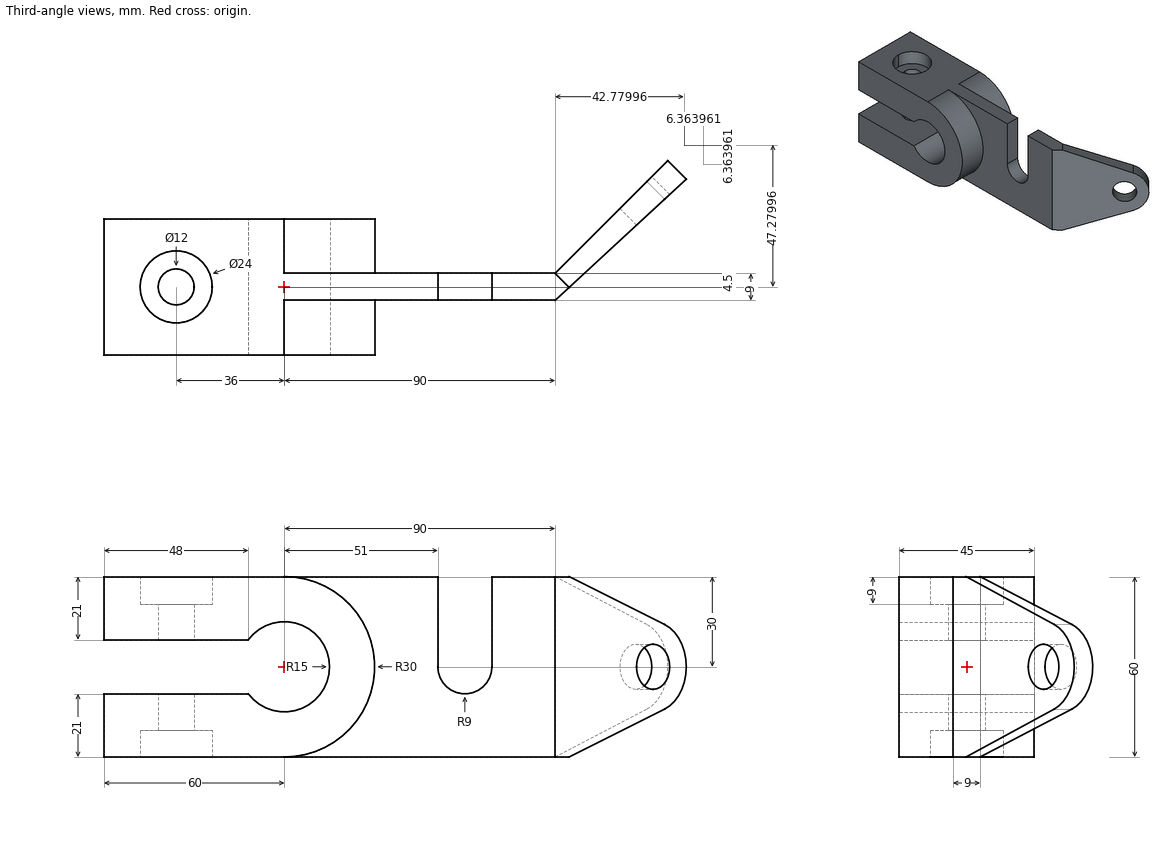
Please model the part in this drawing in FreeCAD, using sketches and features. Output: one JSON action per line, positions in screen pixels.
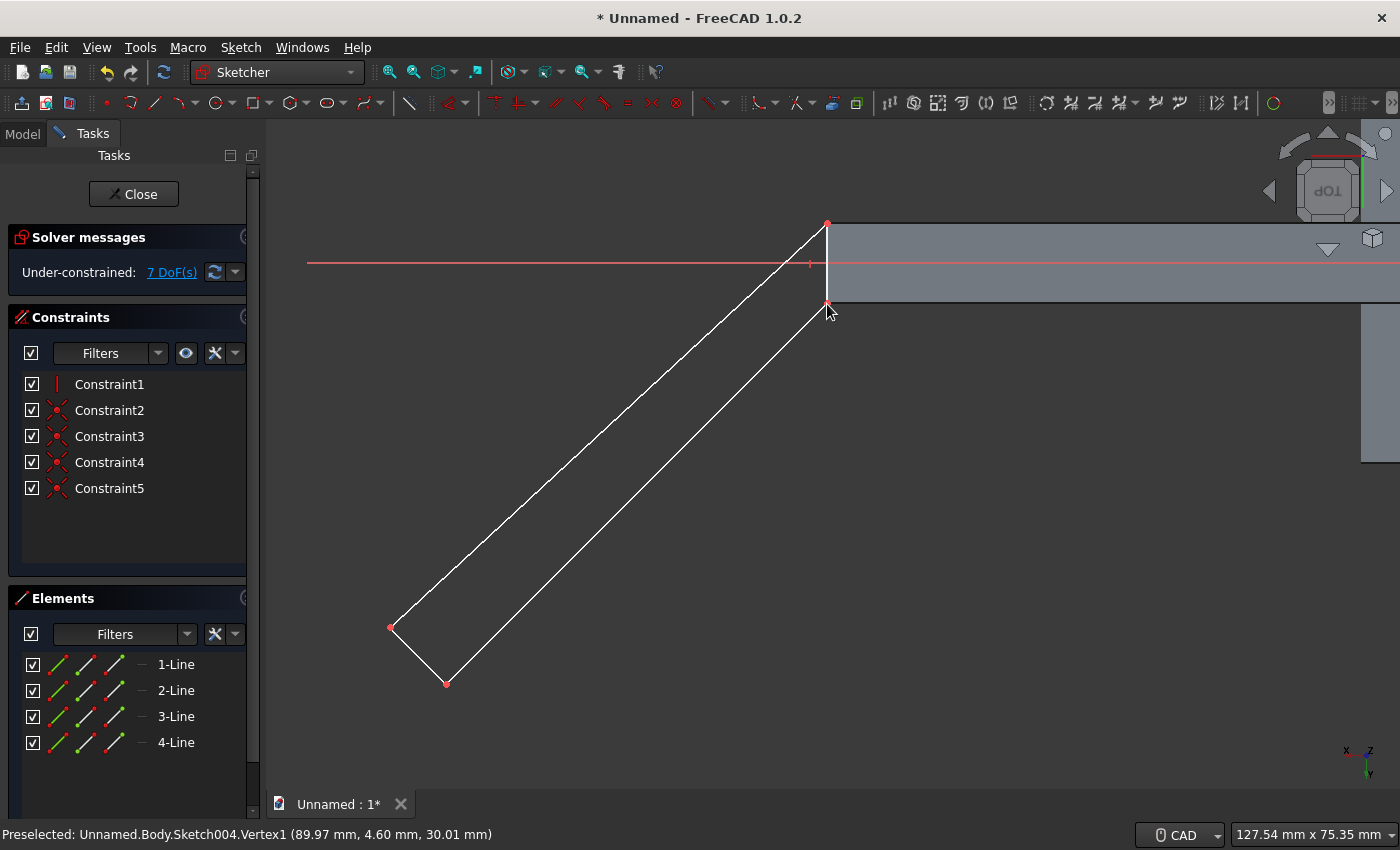
{"action": "left_click", "coordinate": [448, 104]}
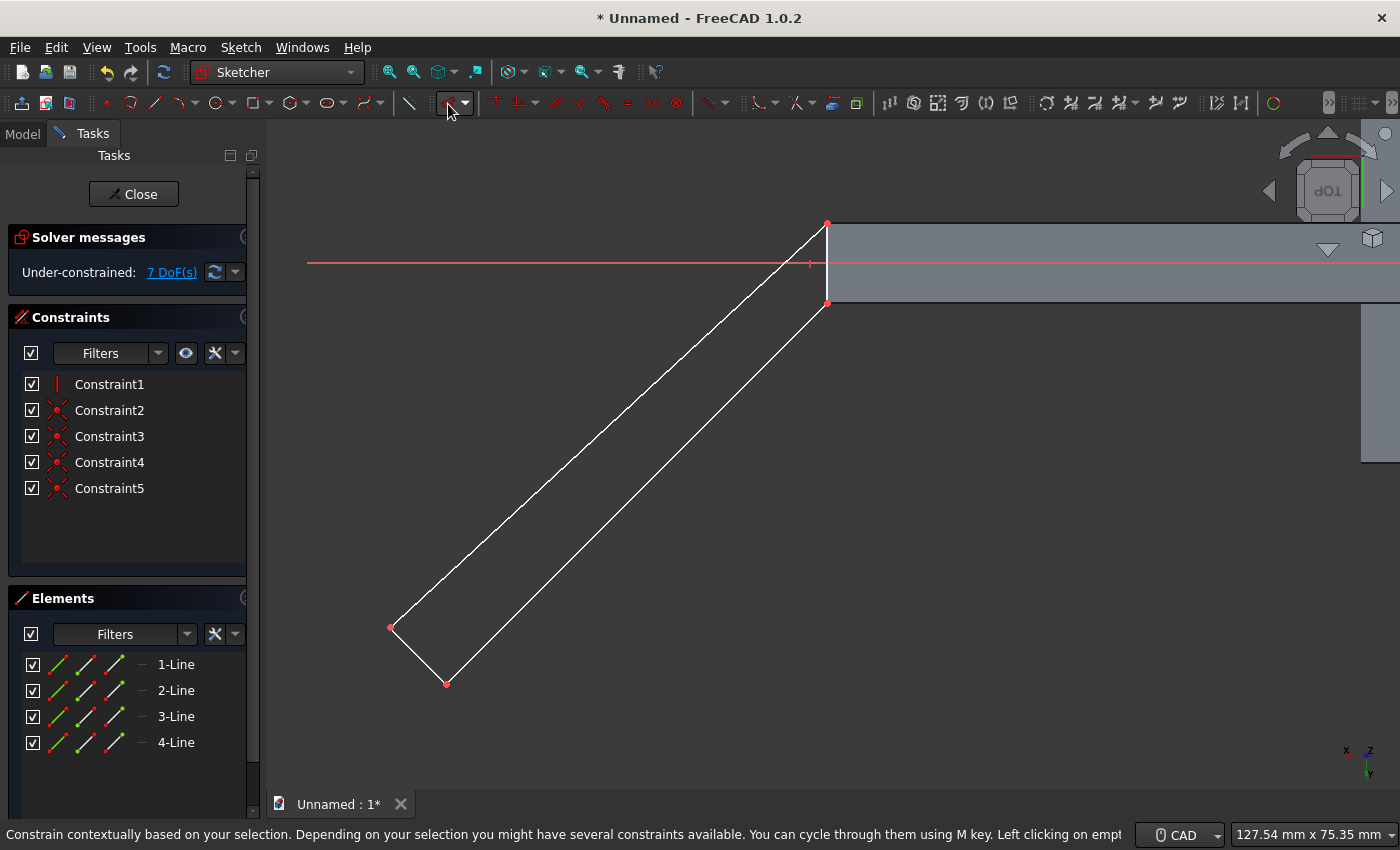
{"action": "left_click", "coordinate": [827, 280]}
{"action": "left_click", "coordinate": [861, 246]}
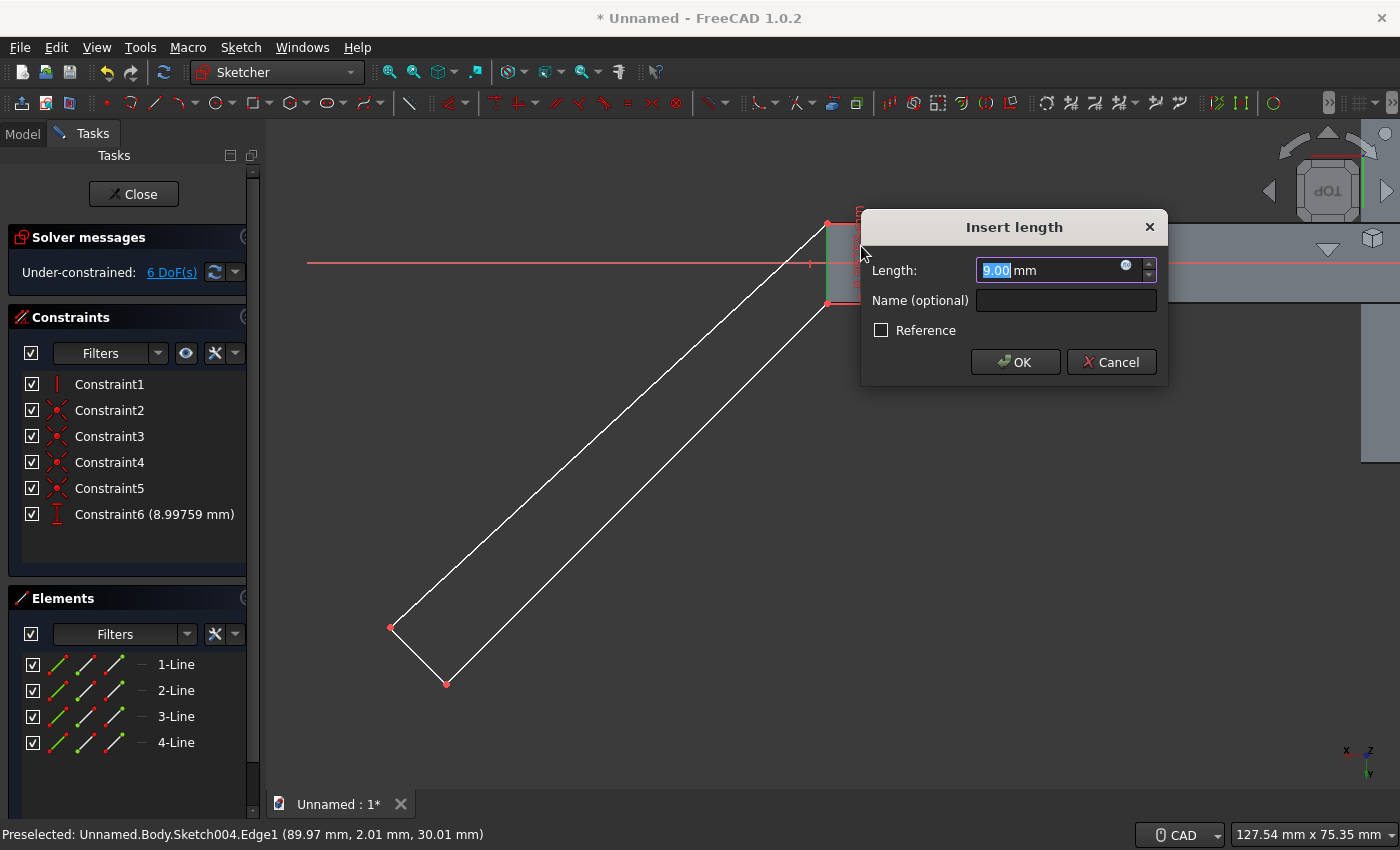
{"action": "type", "text": "9"}
{"action": "key", "text": "Return"}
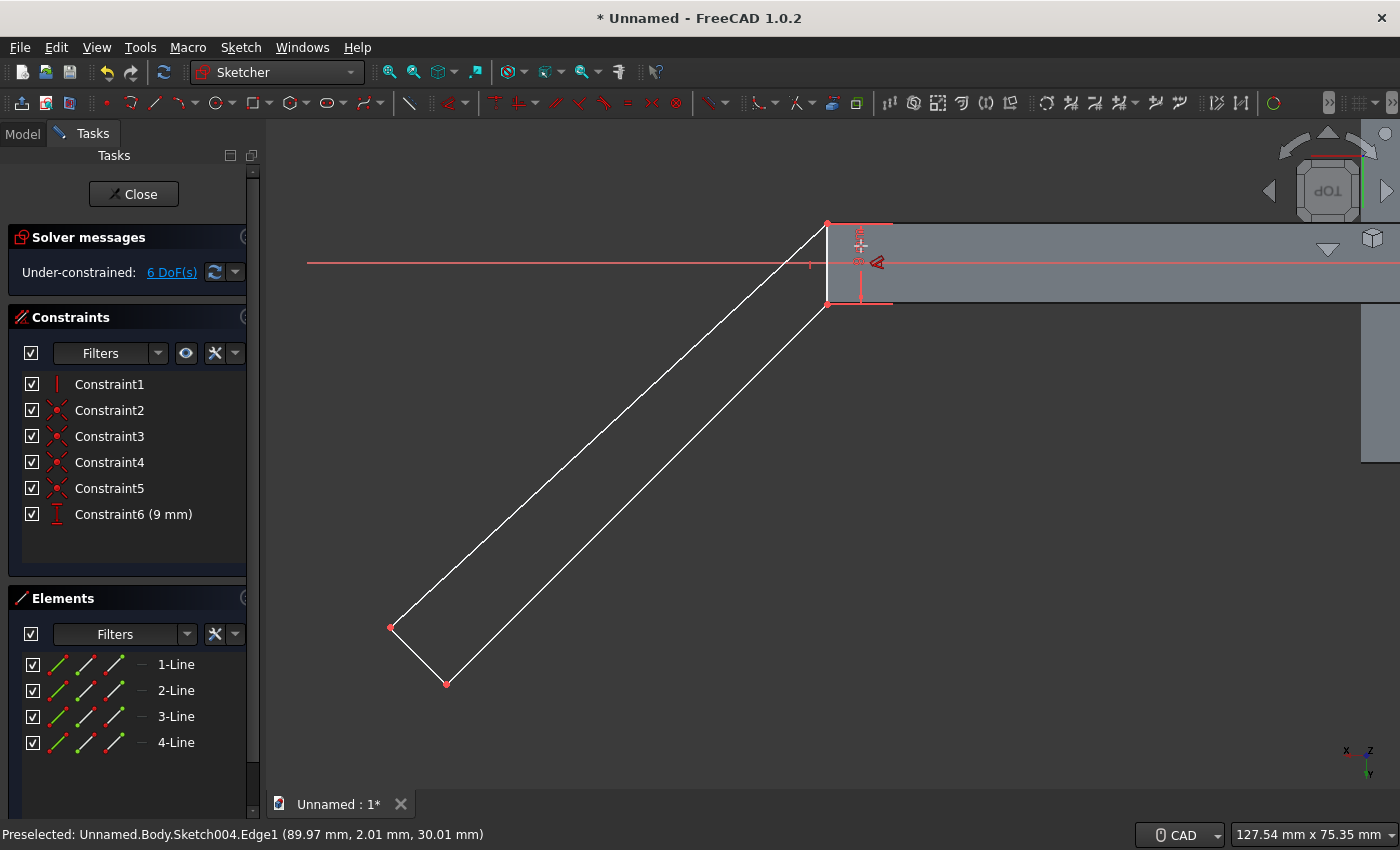
{"action": "left_click", "coordinate": [827, 304]}
{"action": "left_click", "coordinate": [1031, 229]}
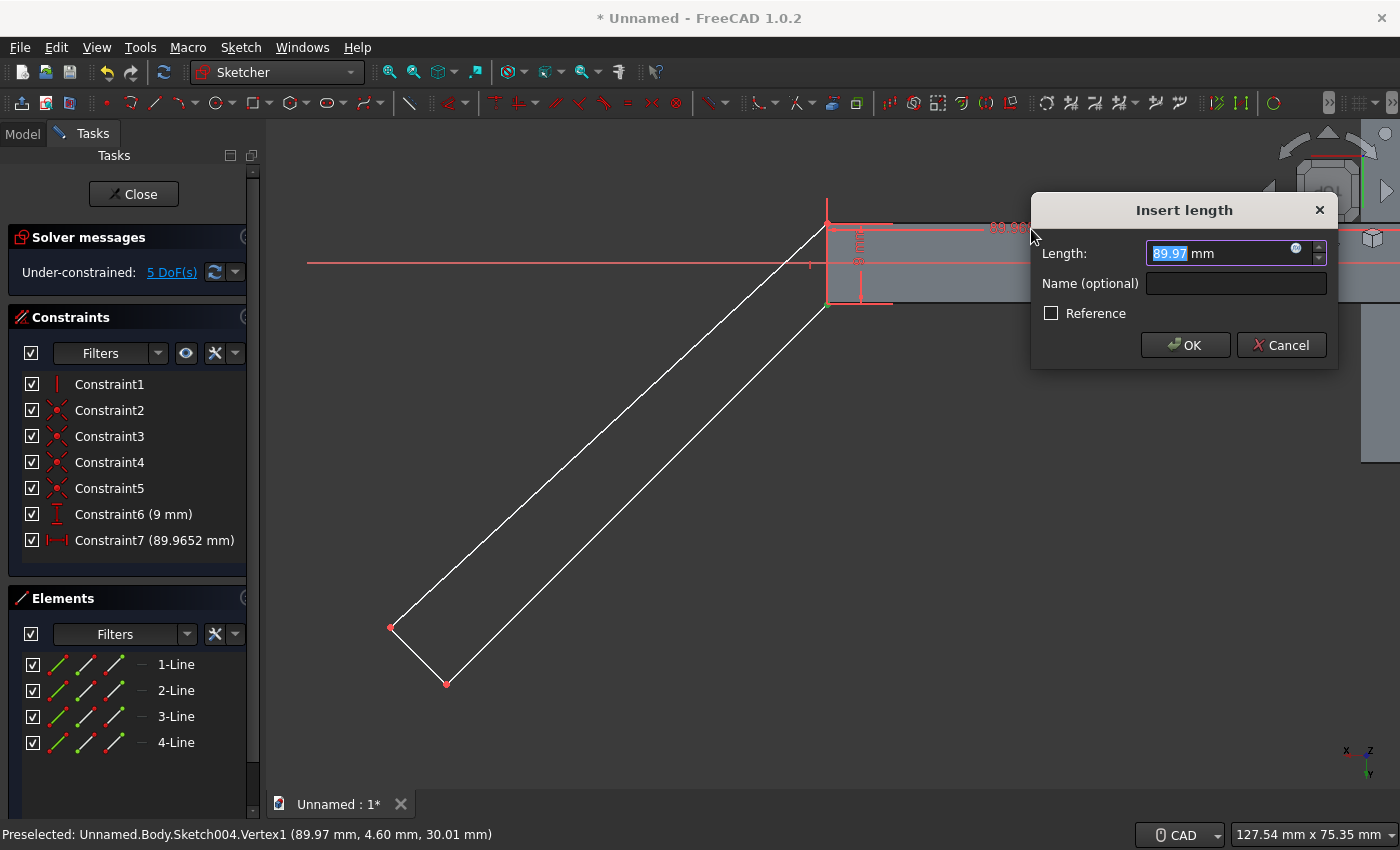
{"action": "type", "text": "90"}
{"action": "key", "text": "Return"}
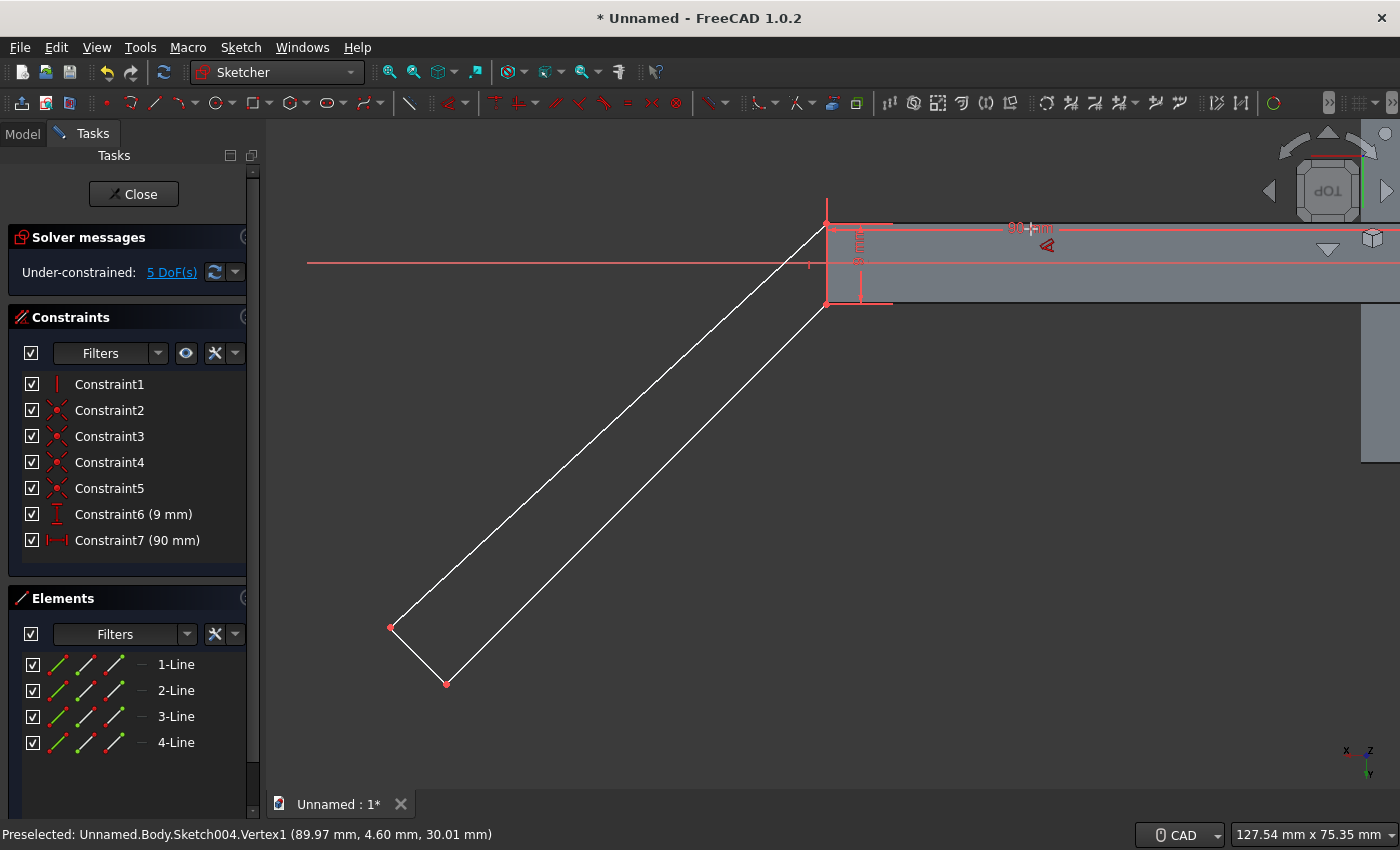
{"action": "left_click", "coordinate": [827, 304]}
{"action": "left_click", "coordinate": [793, 284]}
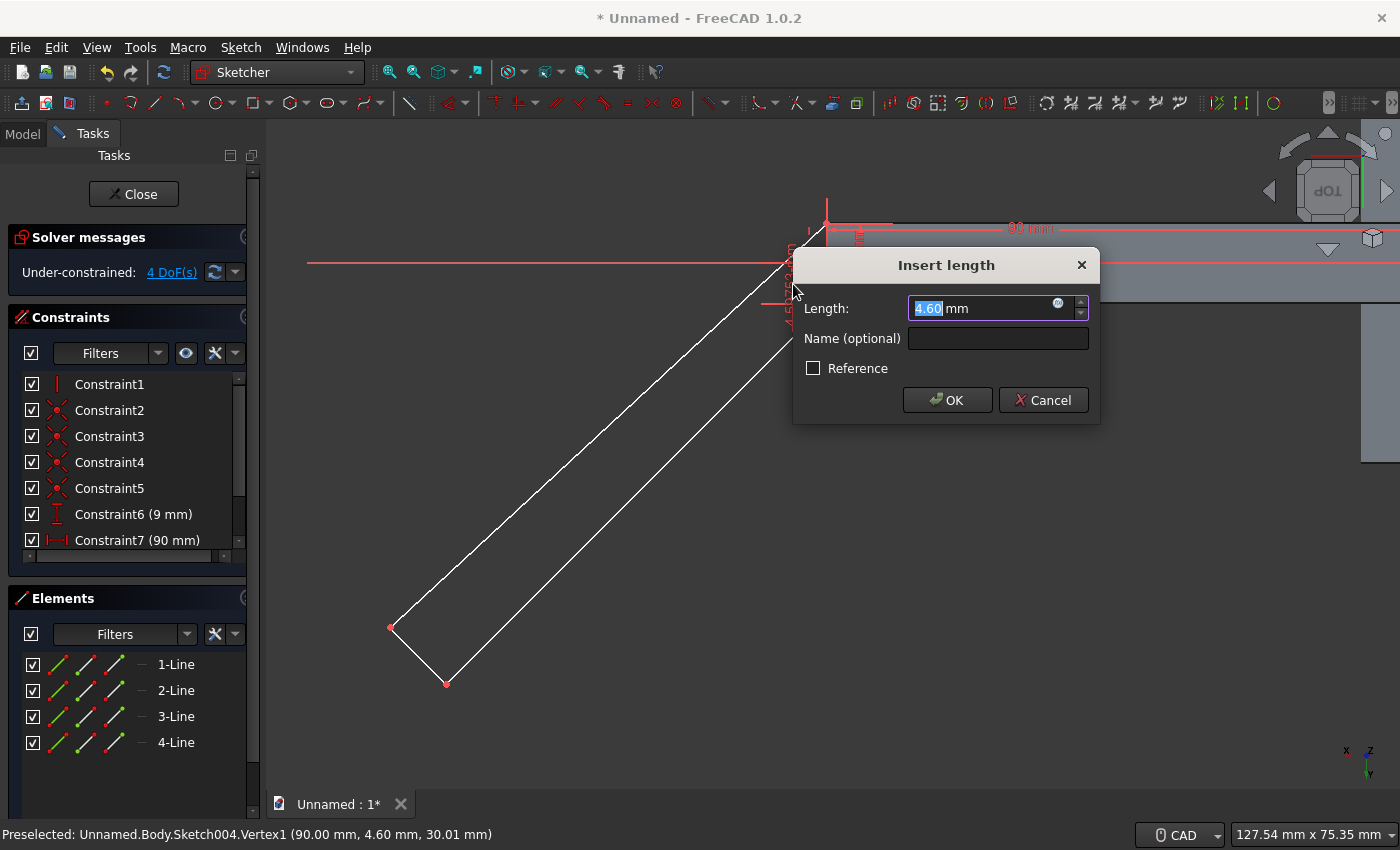
{"action": "type", "text": "4.5"}
{"action": "key", "text": "Return"}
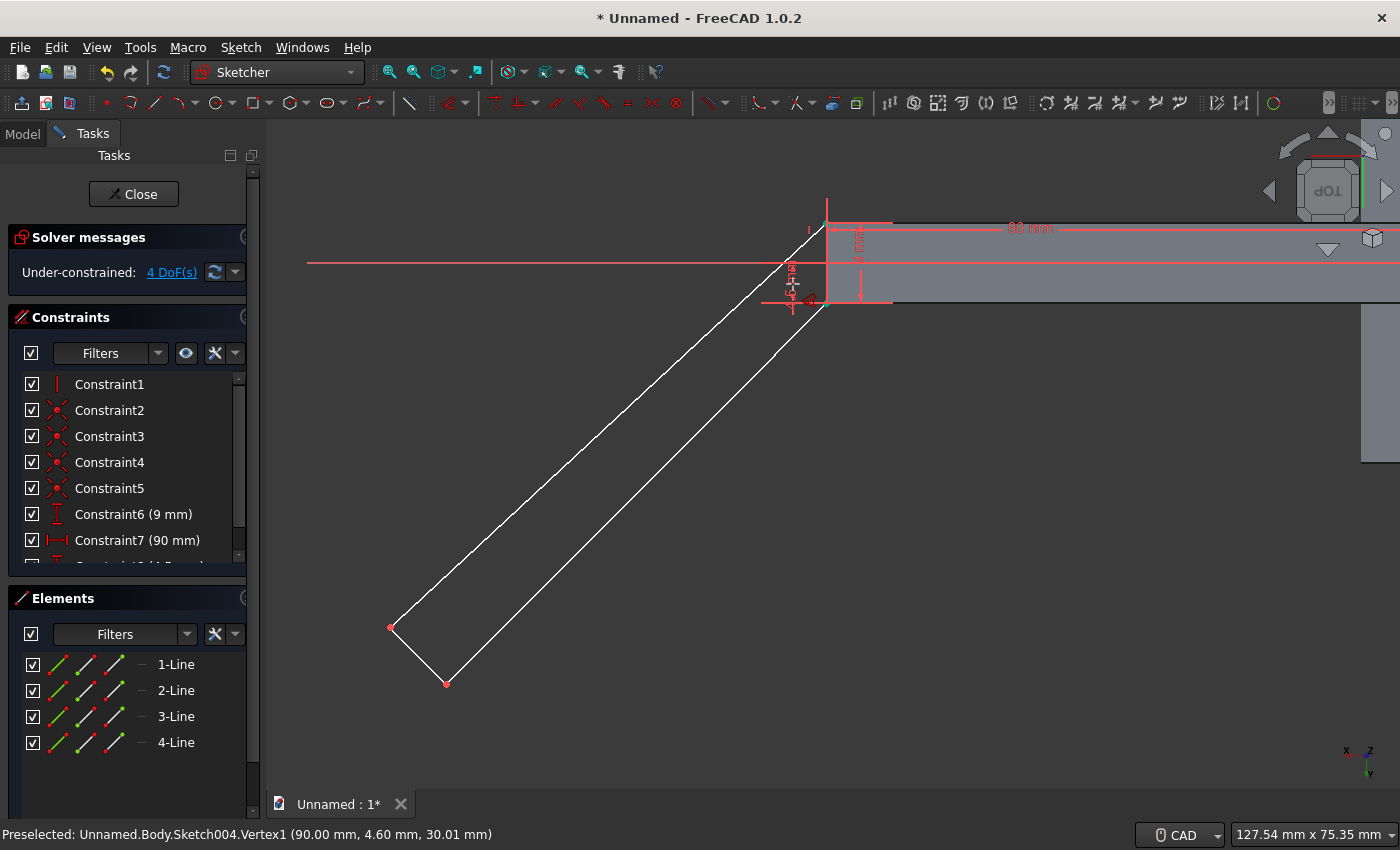
{"action": "left_click", "coordinate": [446, 685]}
{"action": "left_click", "coordinate": [412, 474]}